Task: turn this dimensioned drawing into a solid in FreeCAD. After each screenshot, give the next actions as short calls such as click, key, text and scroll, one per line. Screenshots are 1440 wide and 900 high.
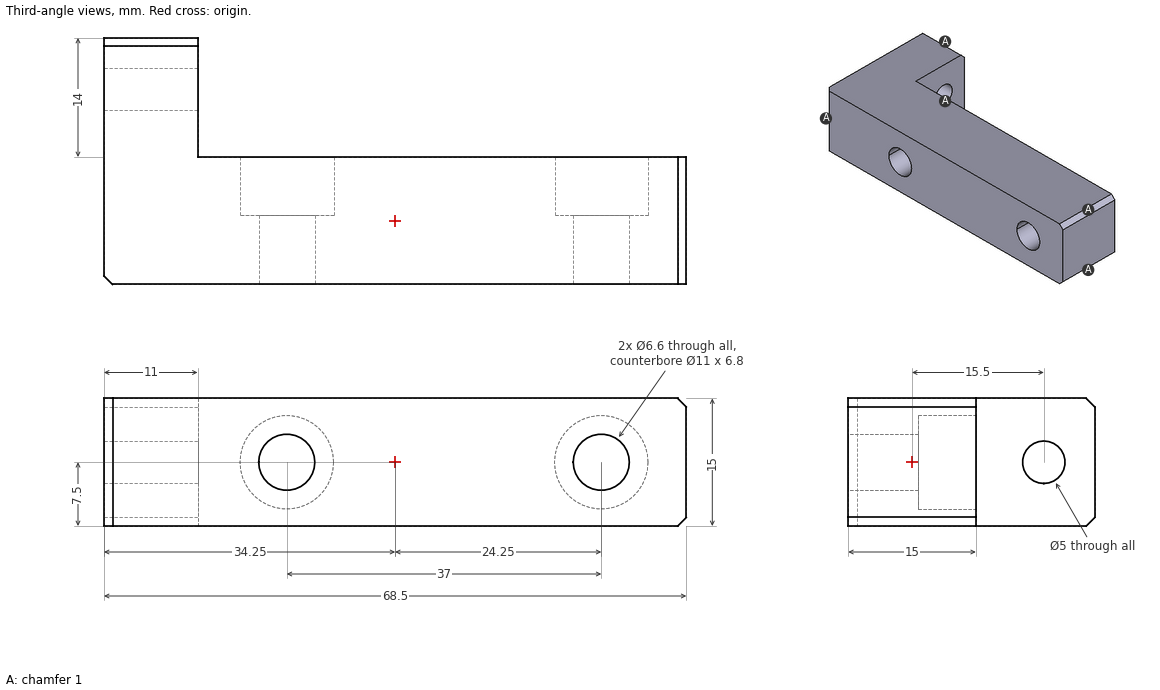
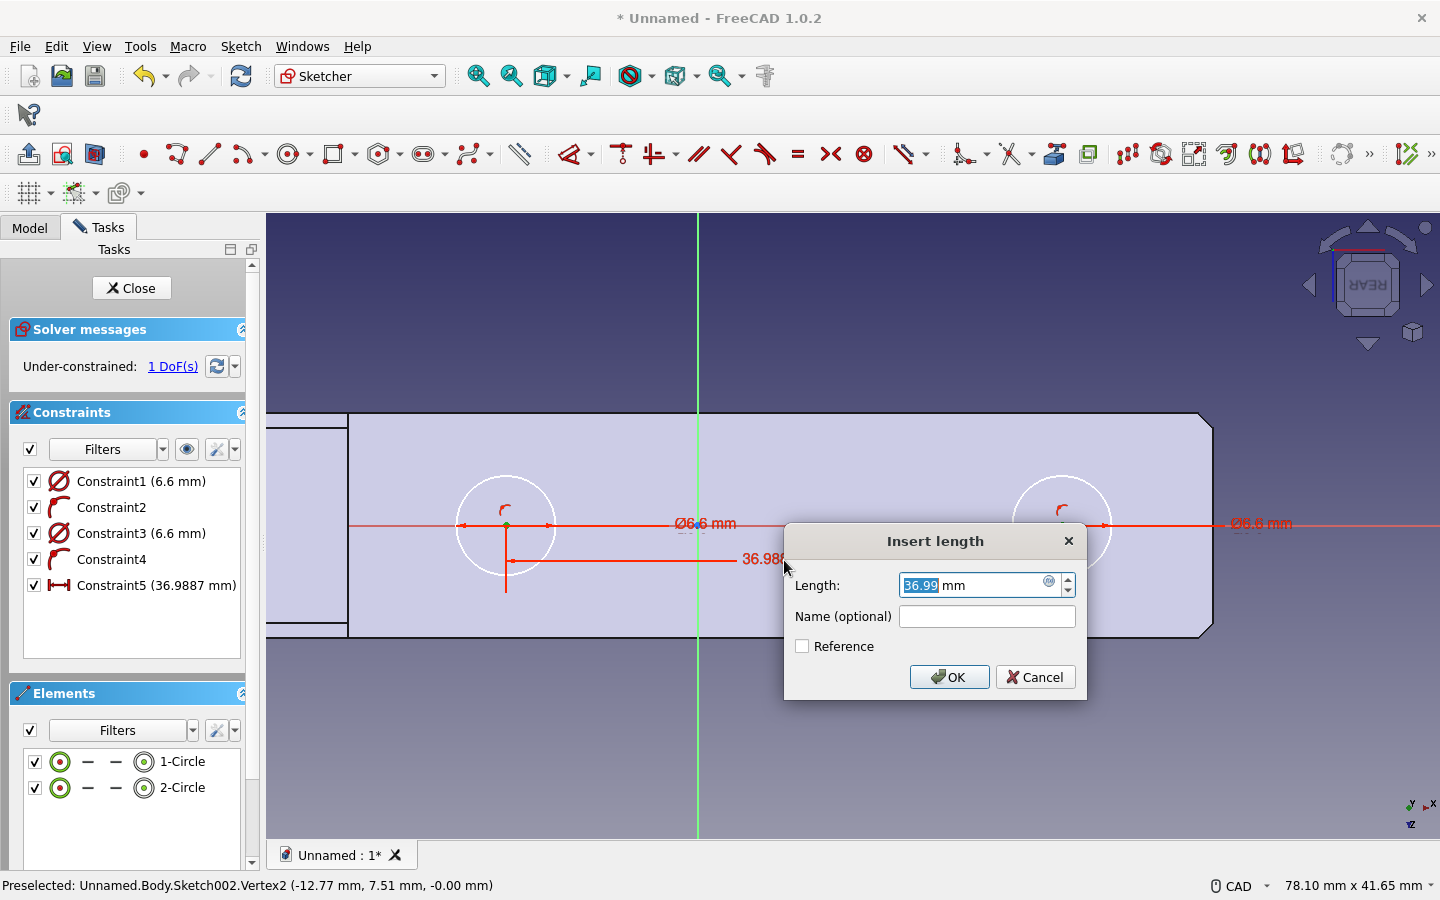
text(37)
key(Return)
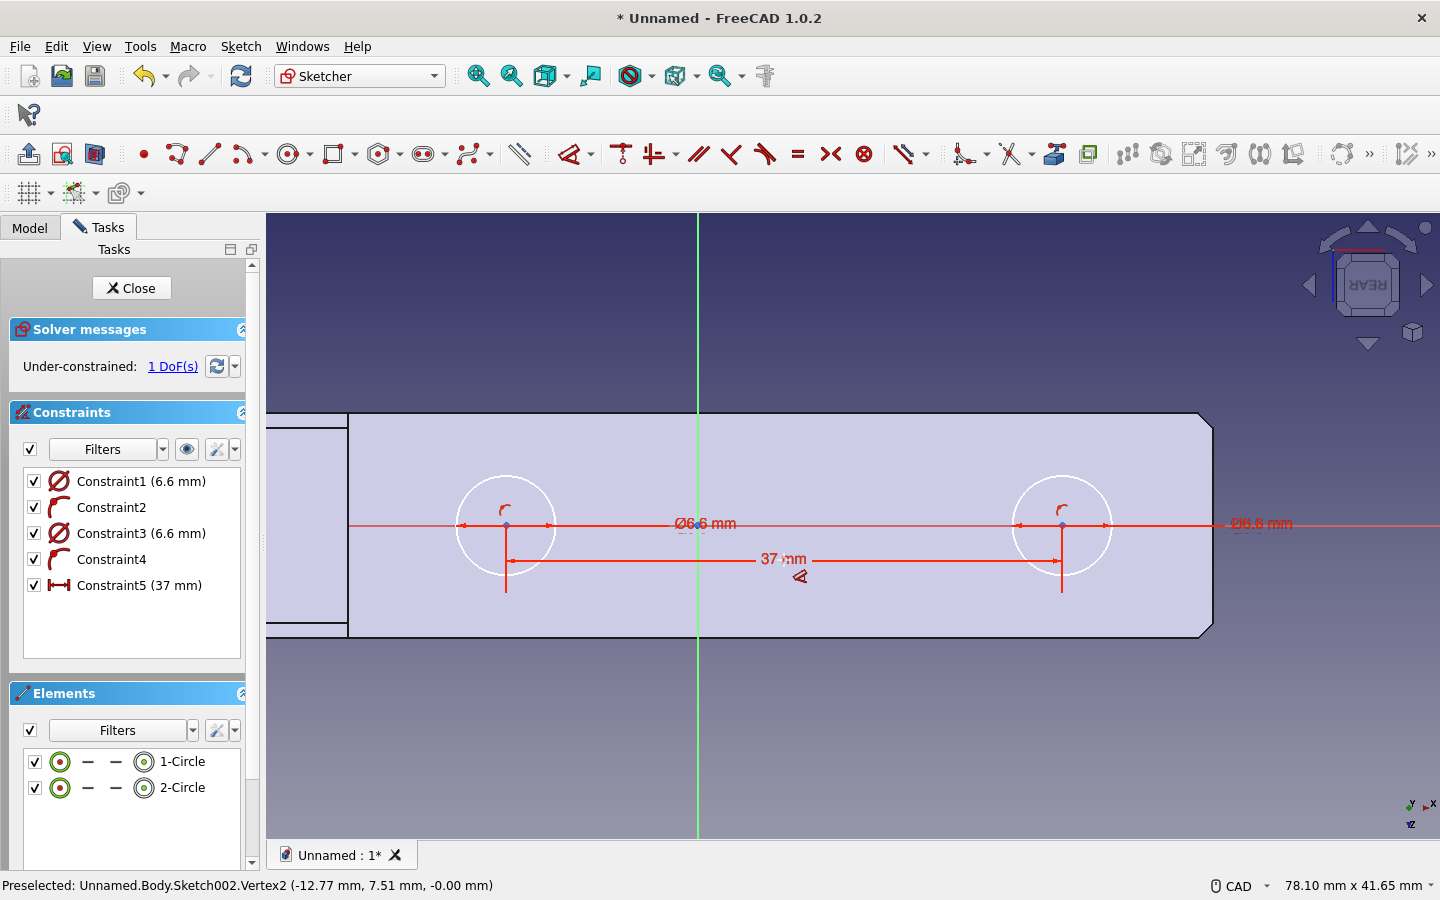
click(1062, 526)
click(880, 560)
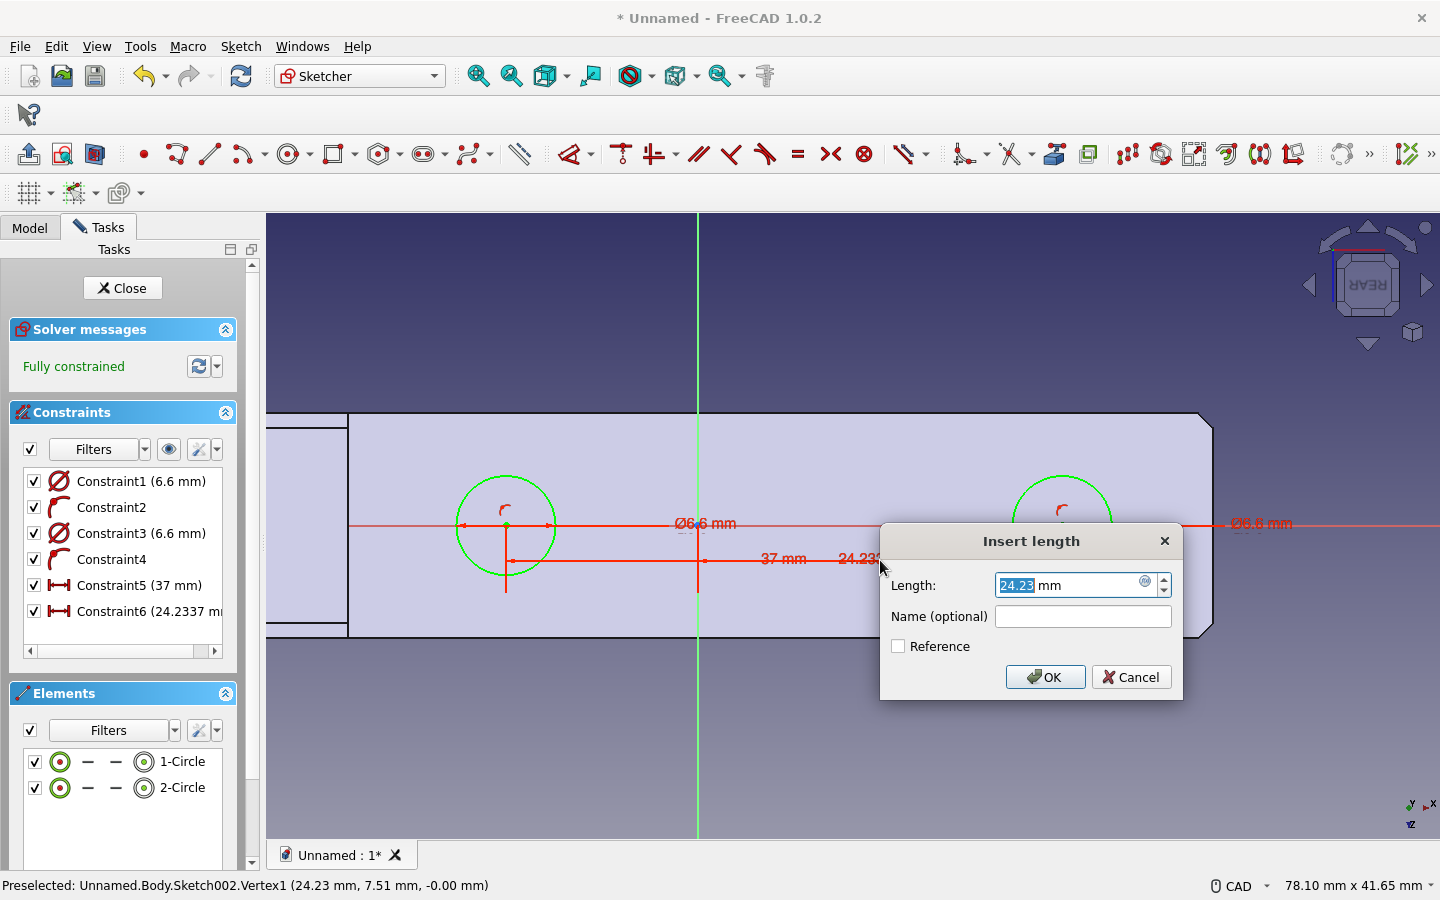
text(24.25)
key(Return)
key(Escape)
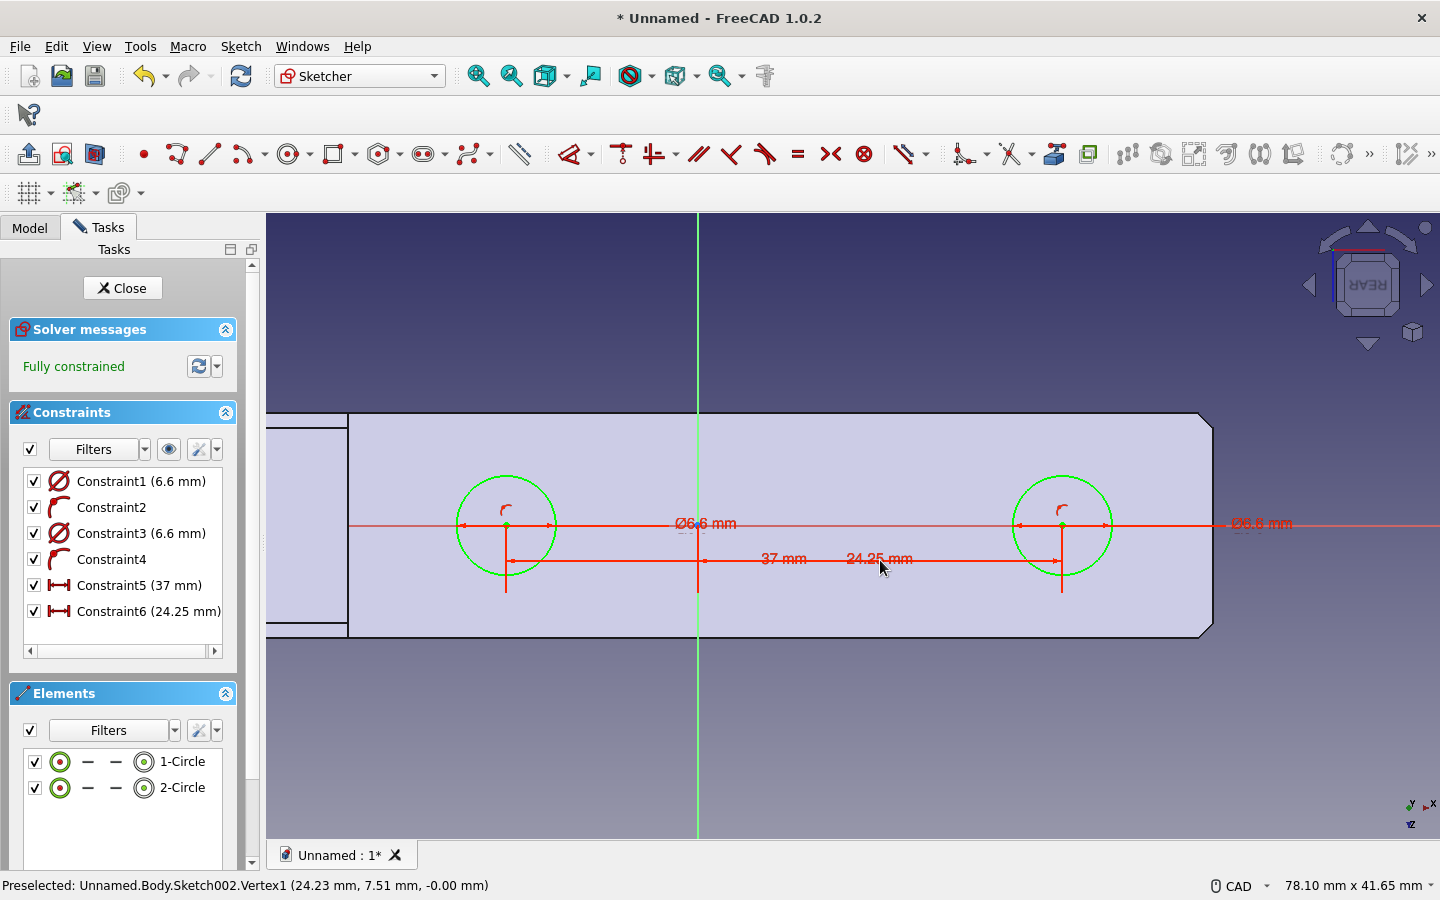
click(123, 288)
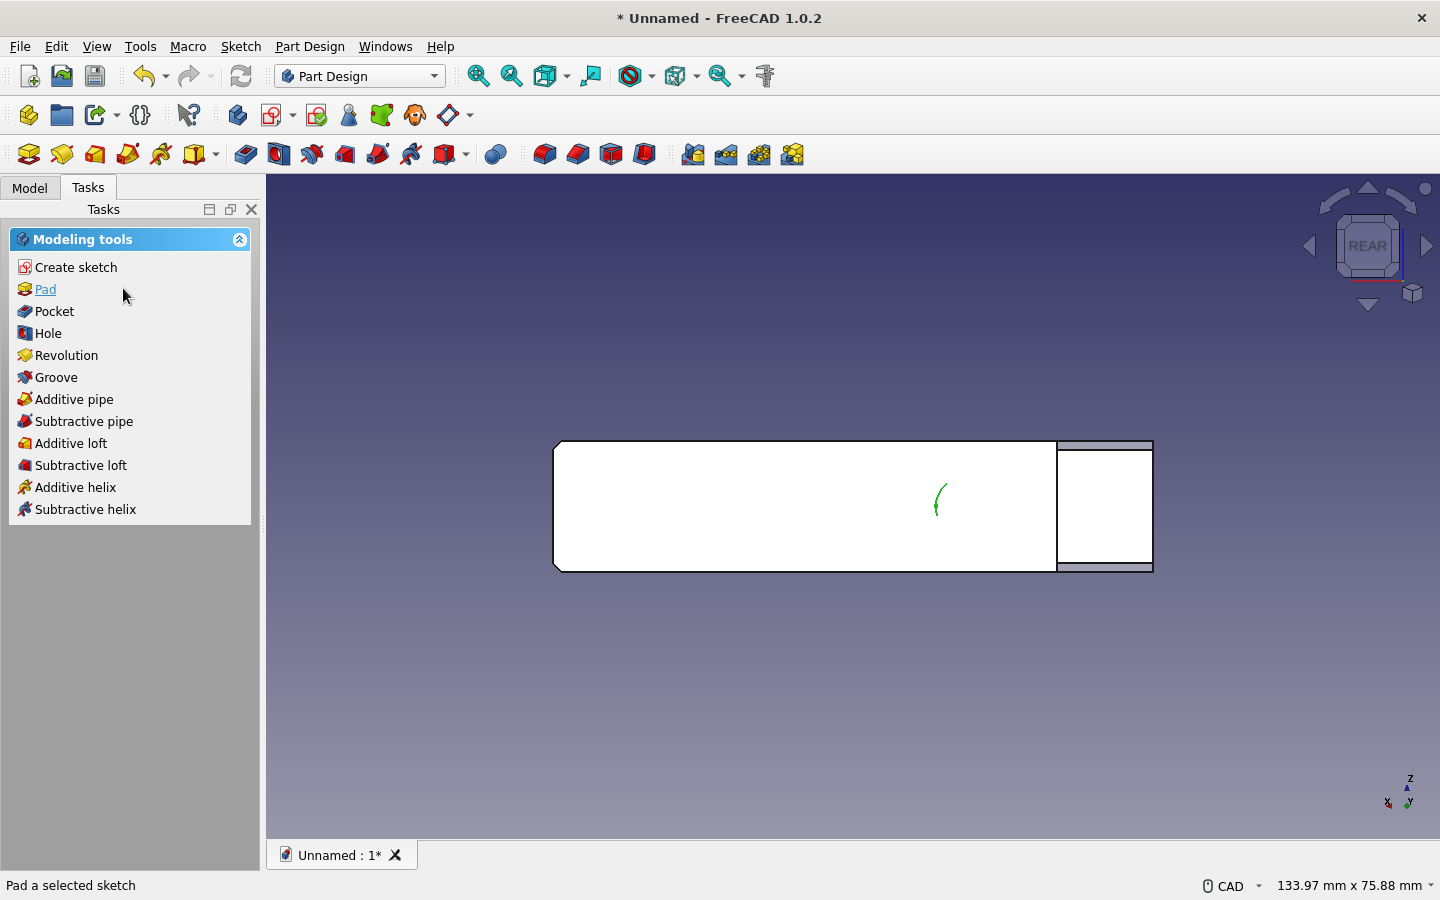
click(279, 154)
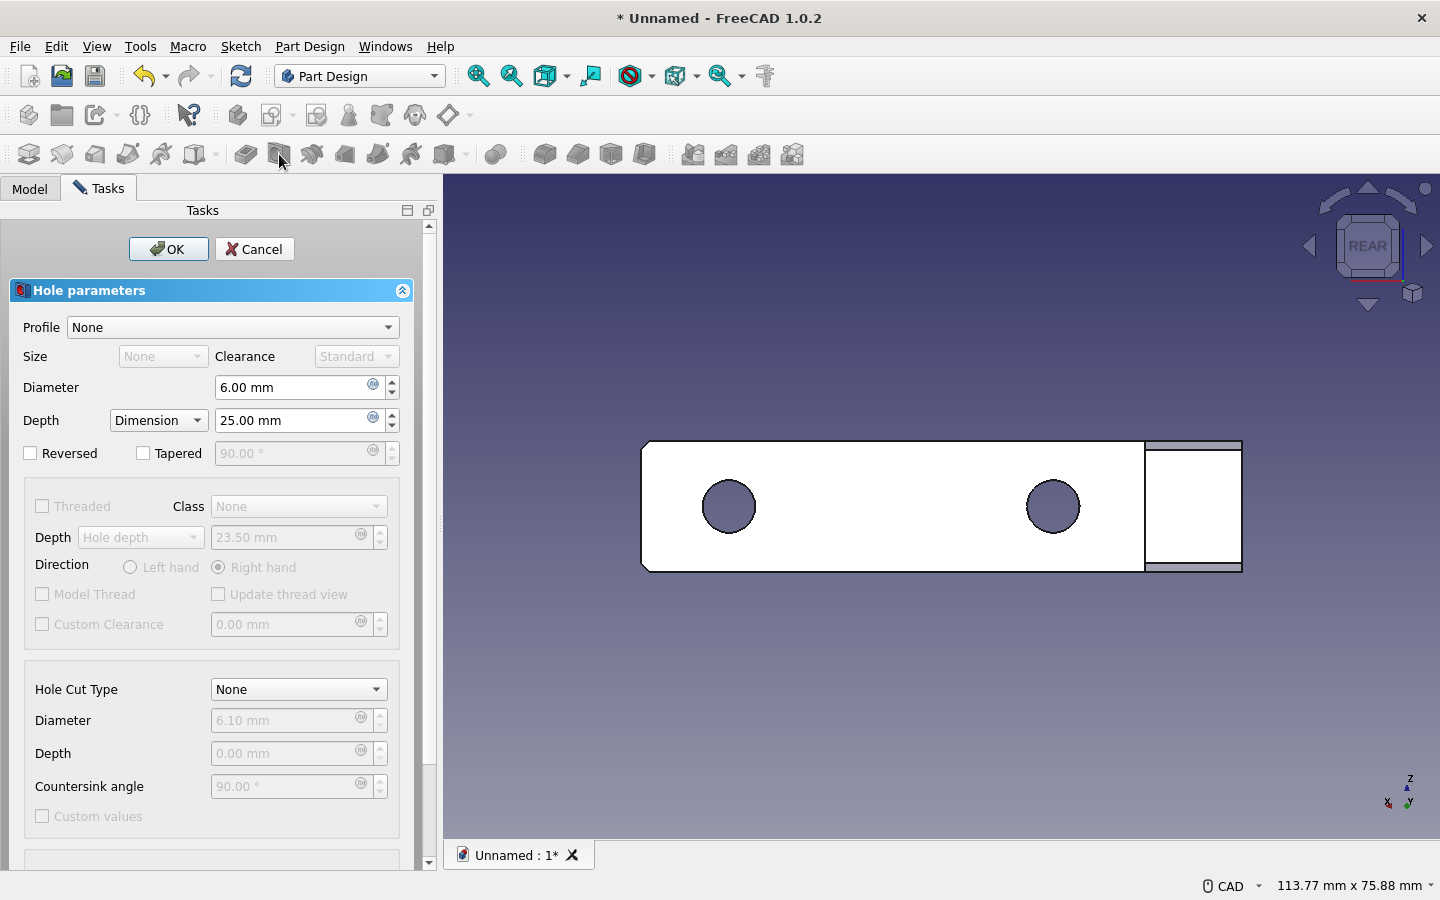
triple_click(300, 388)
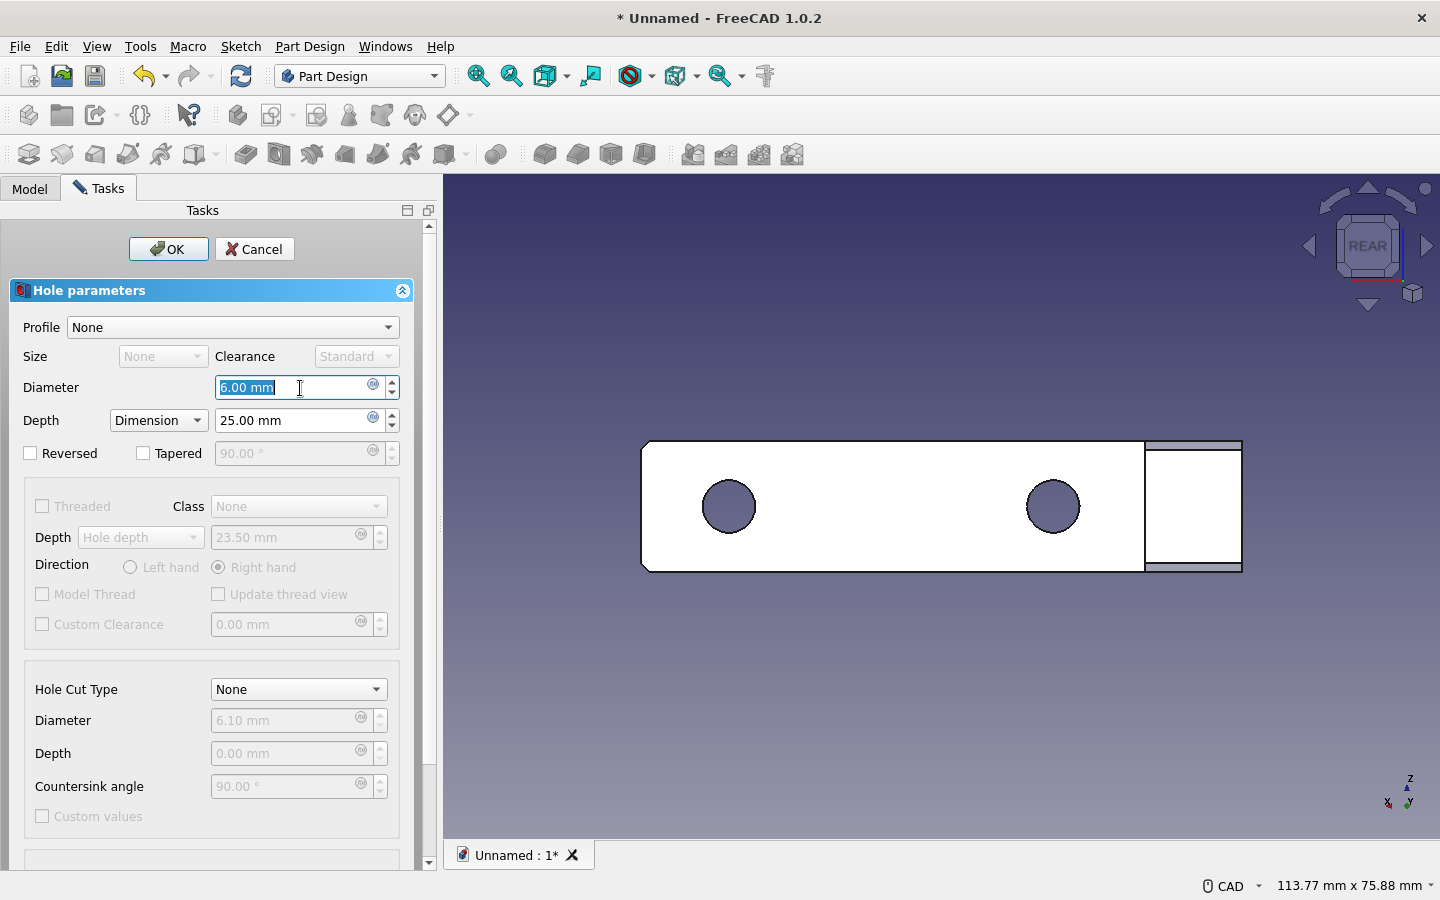
text(6.6)
key(Tab)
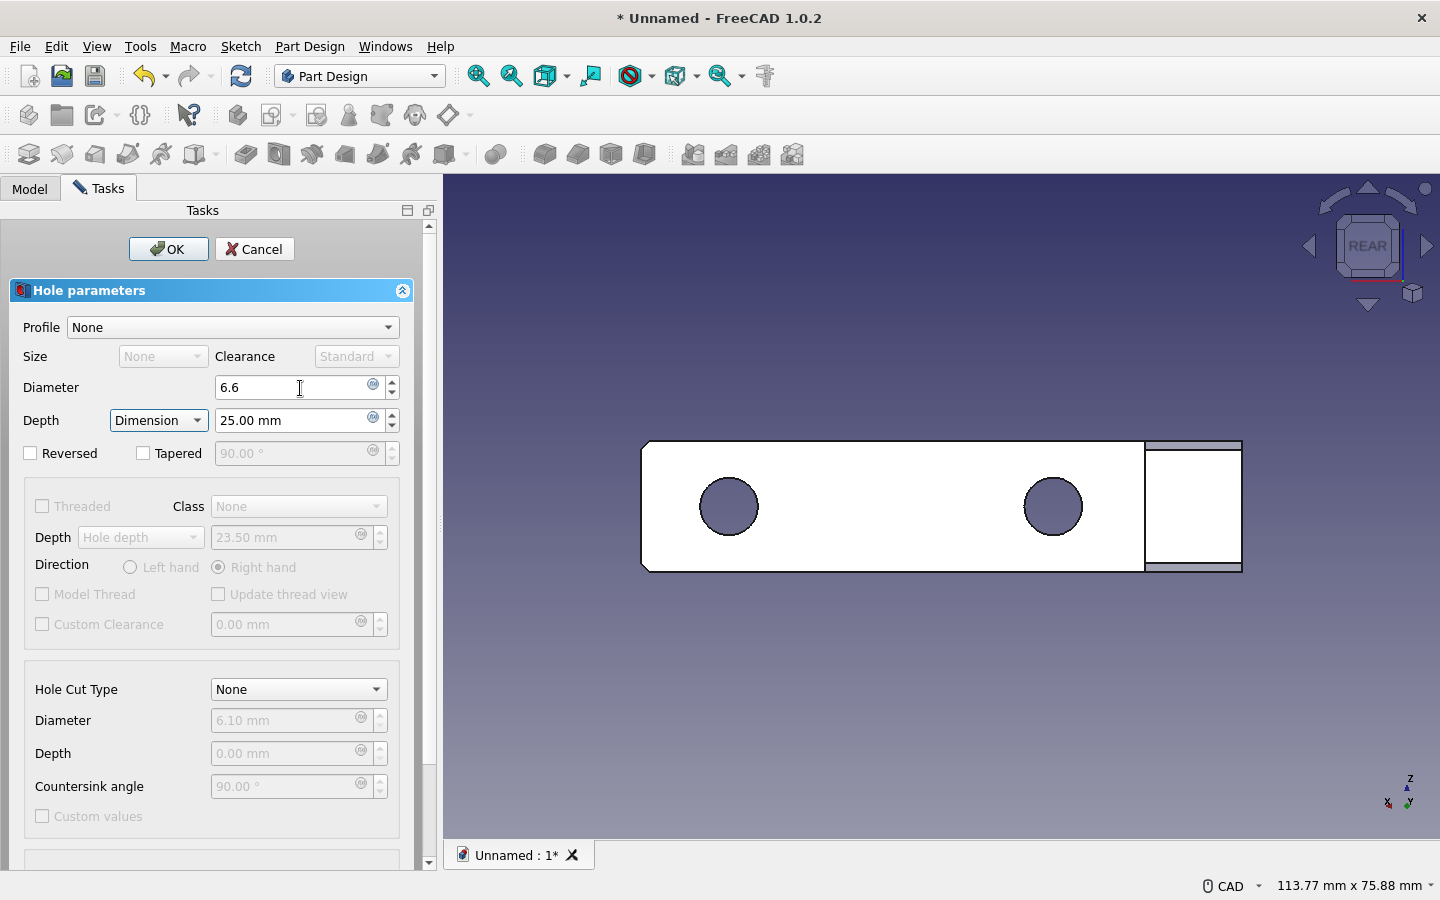
click(160, 420)